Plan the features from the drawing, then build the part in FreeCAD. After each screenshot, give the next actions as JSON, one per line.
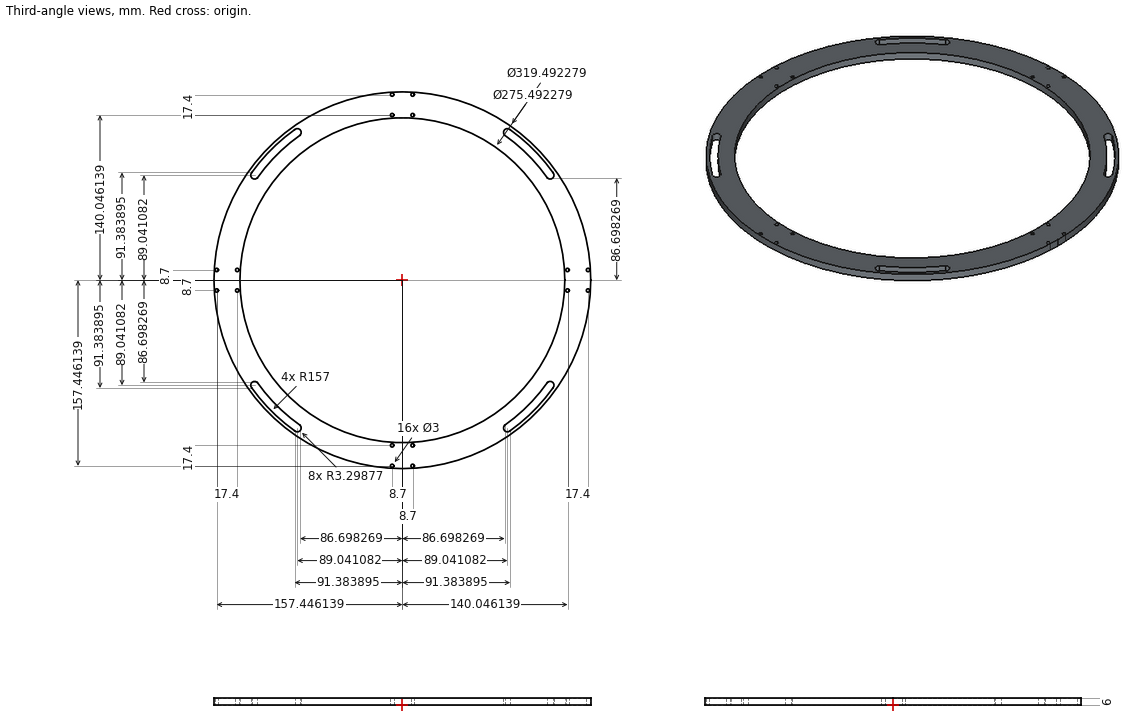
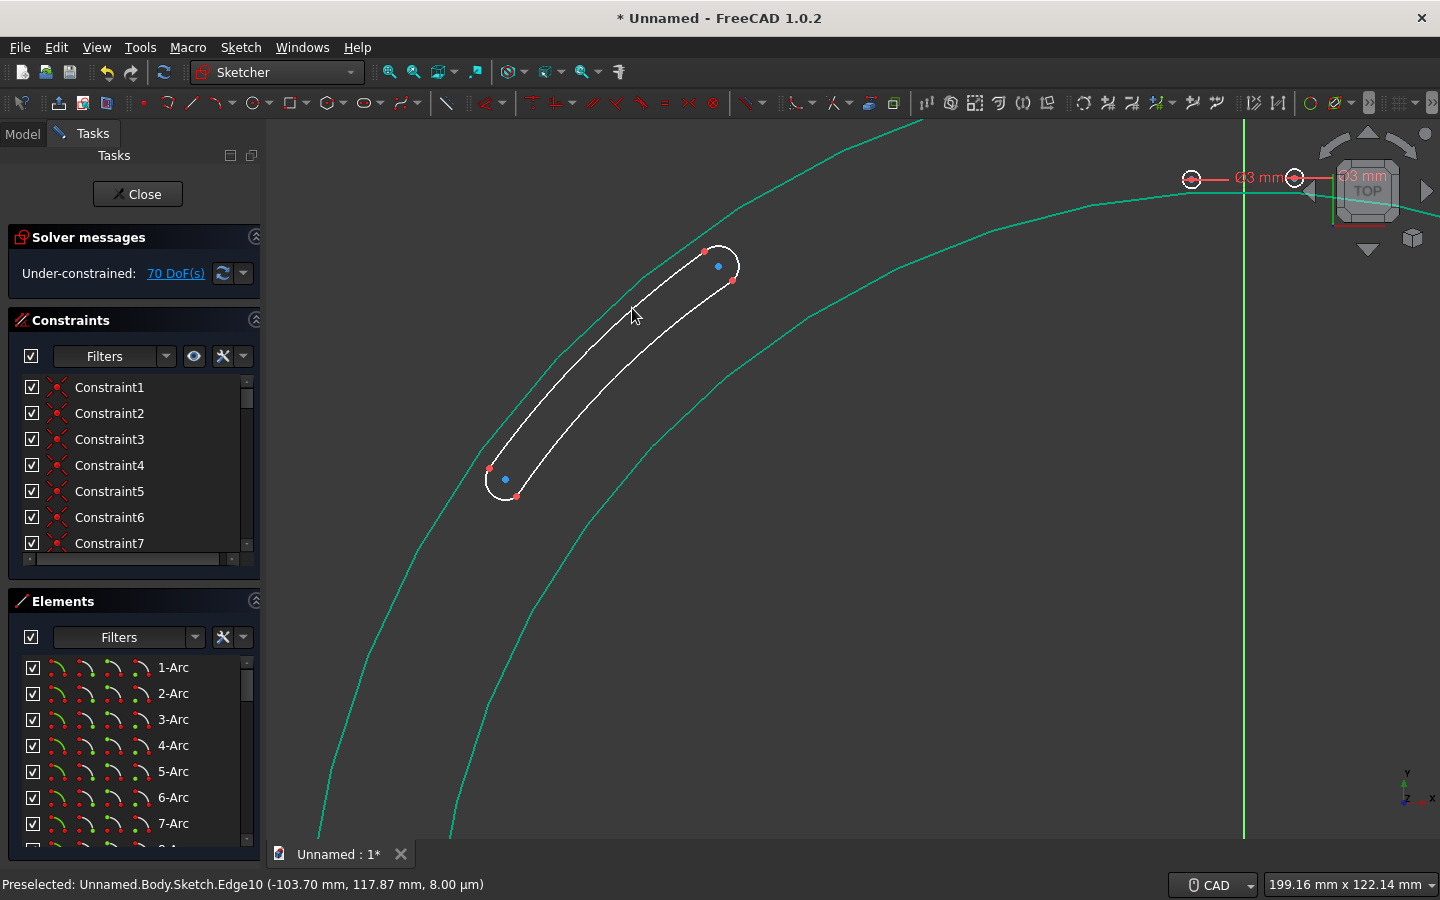
{"action": "left_click", "coordinate": [576, 339]}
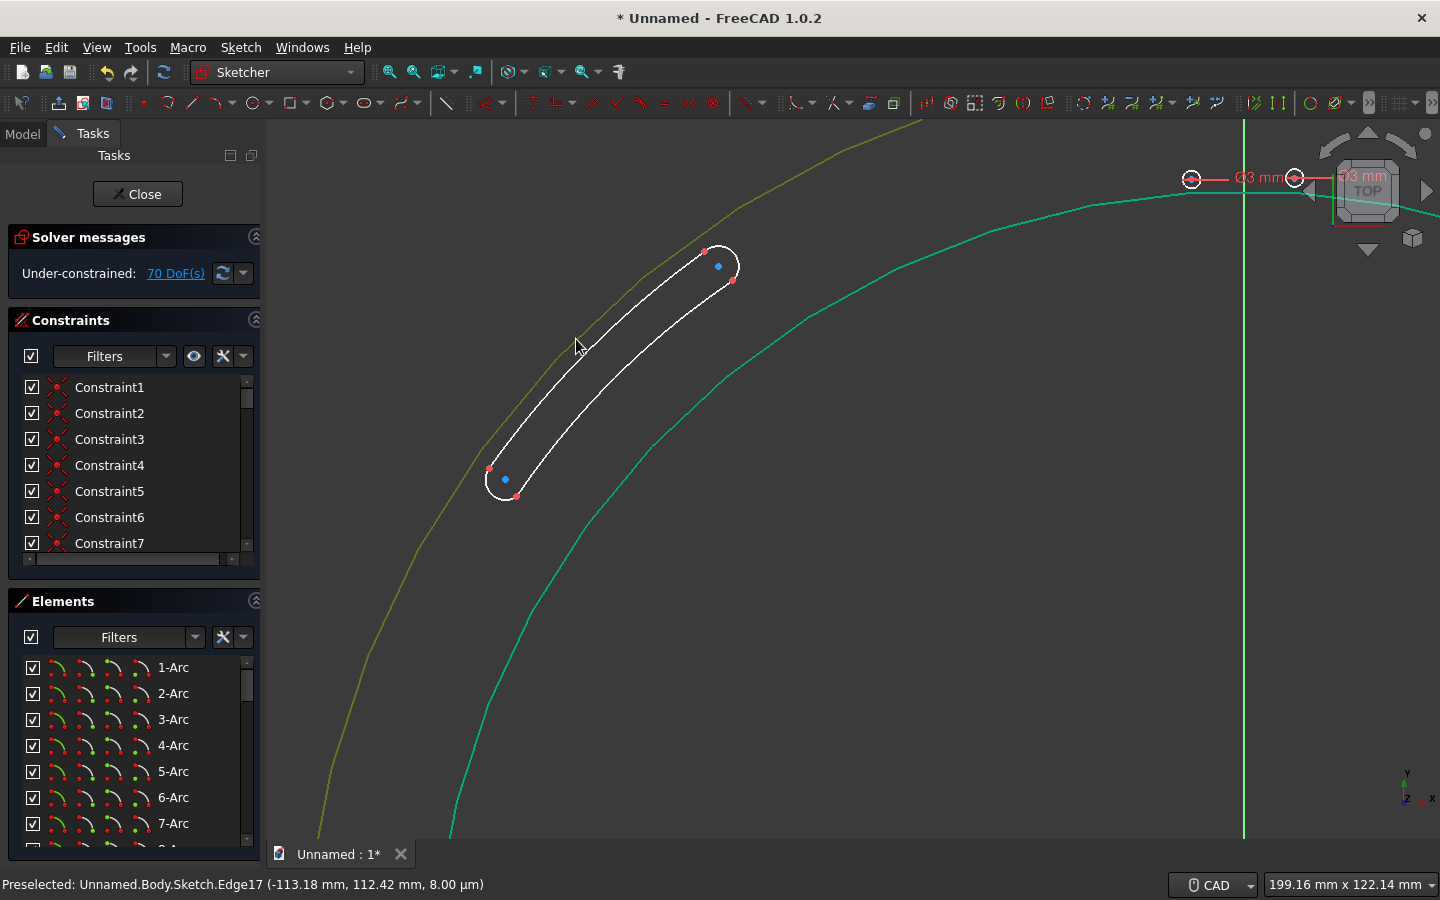
{"action": "left_click", "coordinate": [659, 337]}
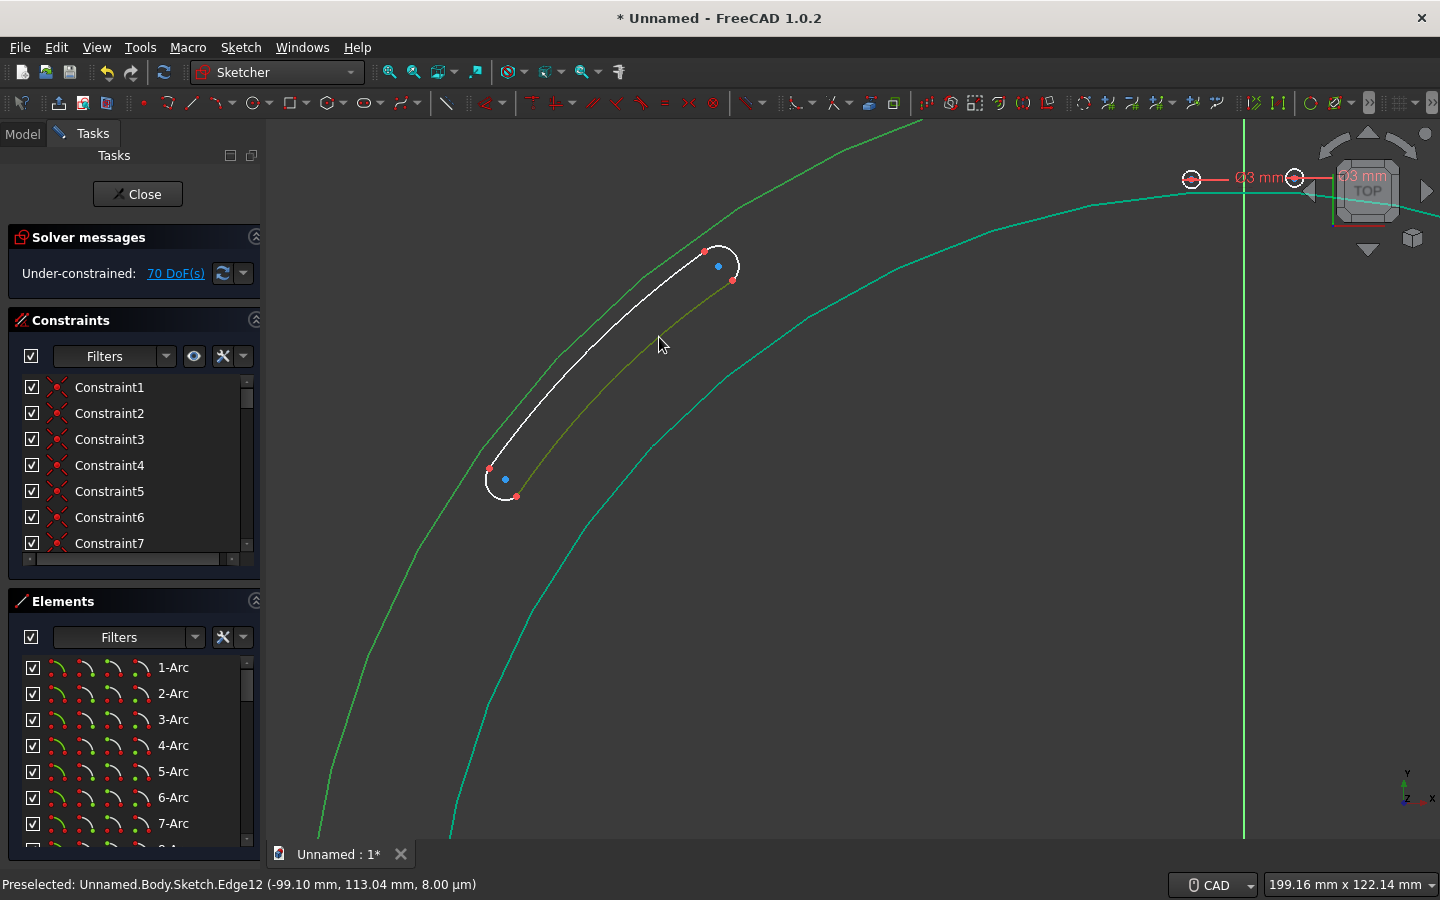
{"action": "left_click", "coordinate": [532, 104]}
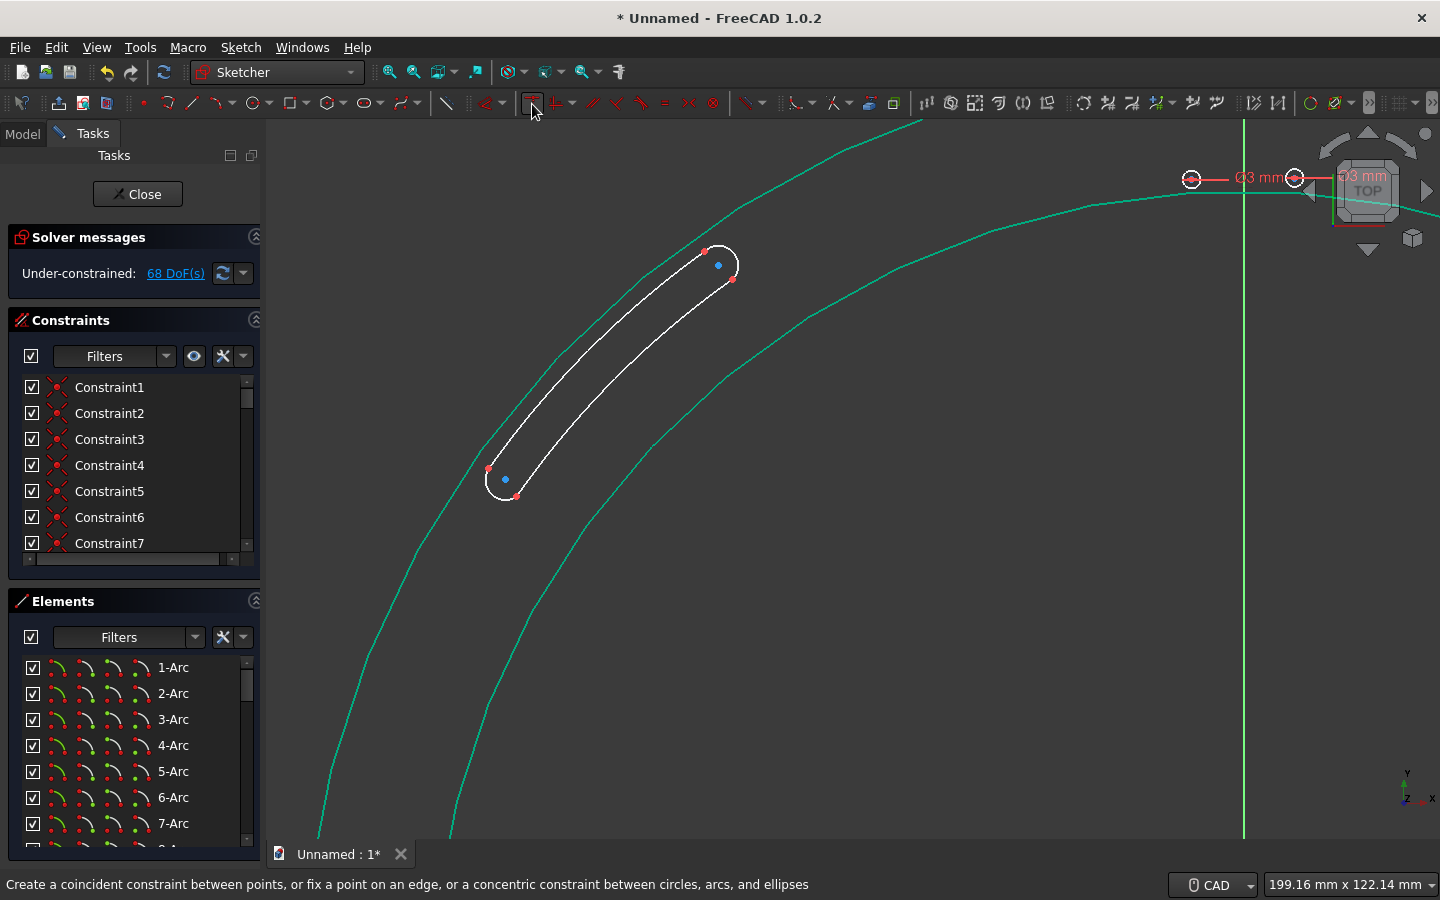
{"action": "left_click", "coordinate": [576, 339]}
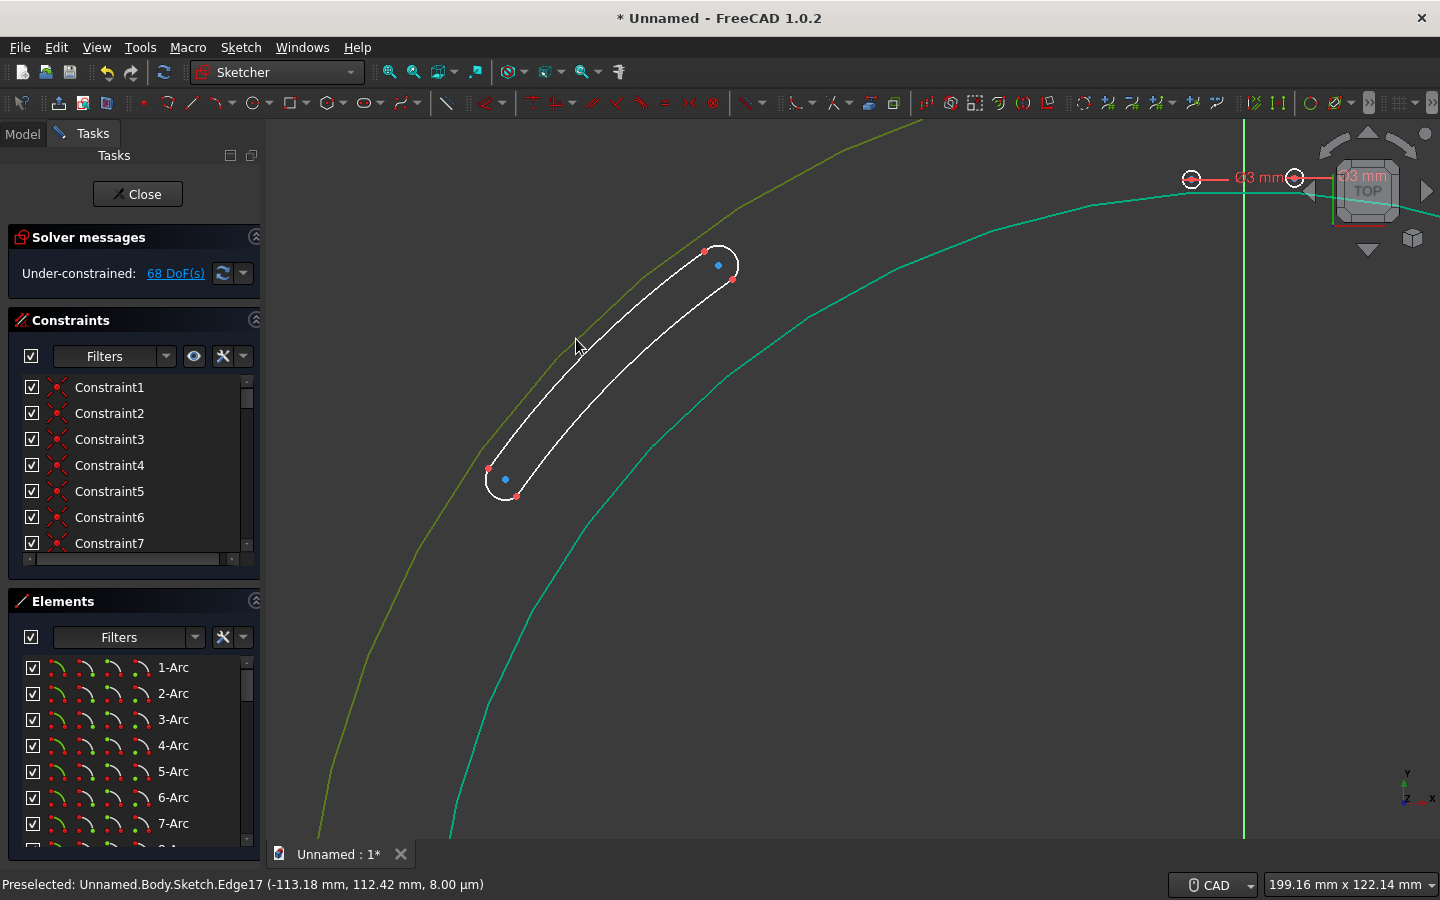
{"action": "scroll", "coordinate": [634, 307], "scroll_direction": "down", "scroll_amount": 7}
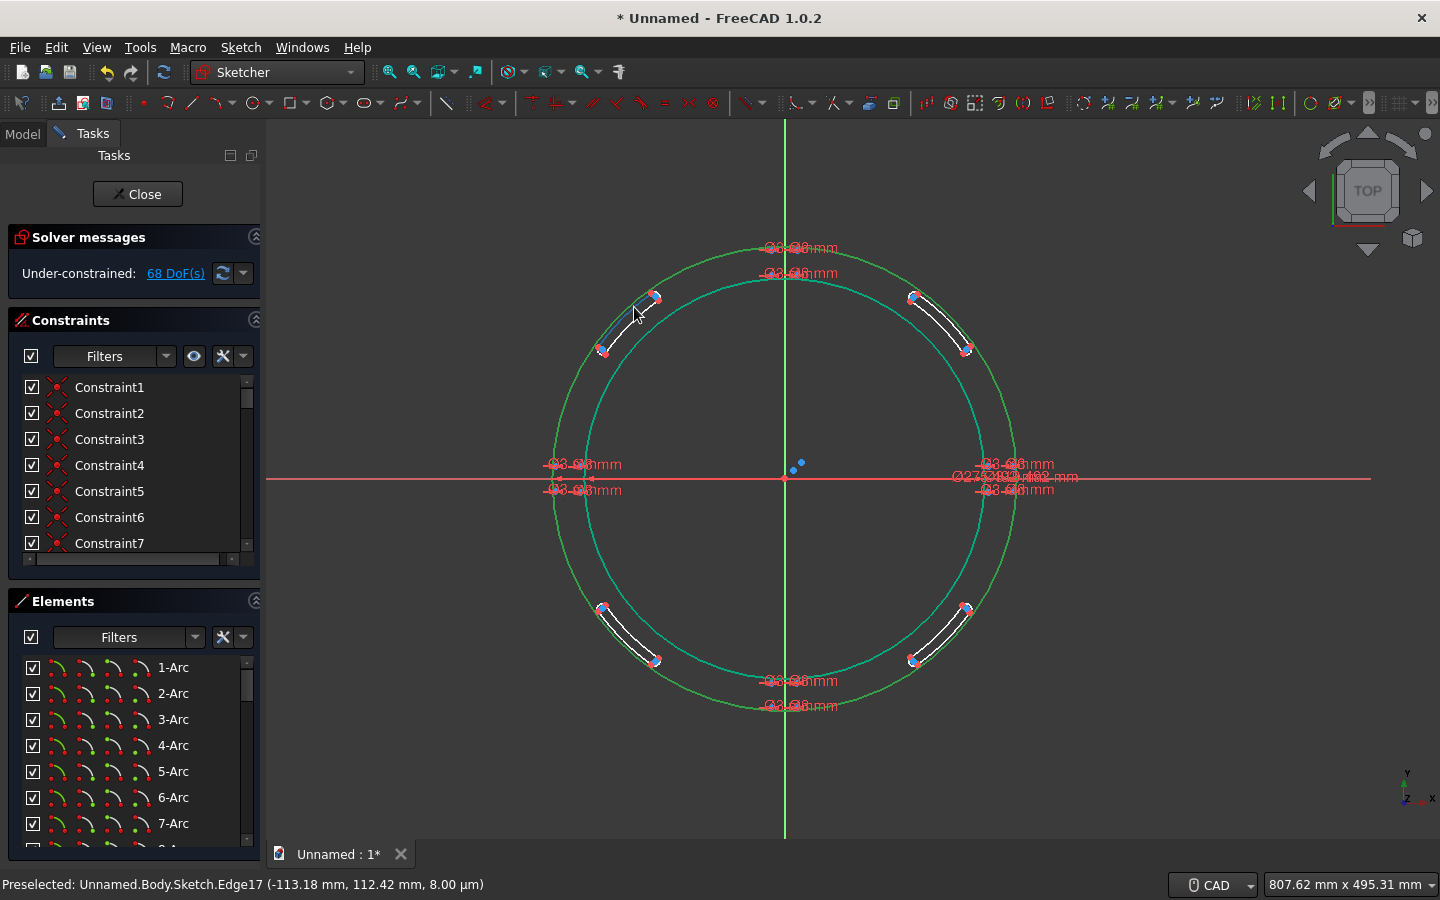
{"action": "scroll", "coordinate": [956, 329], "scroll_direction": "up", "scroll_amount": 7}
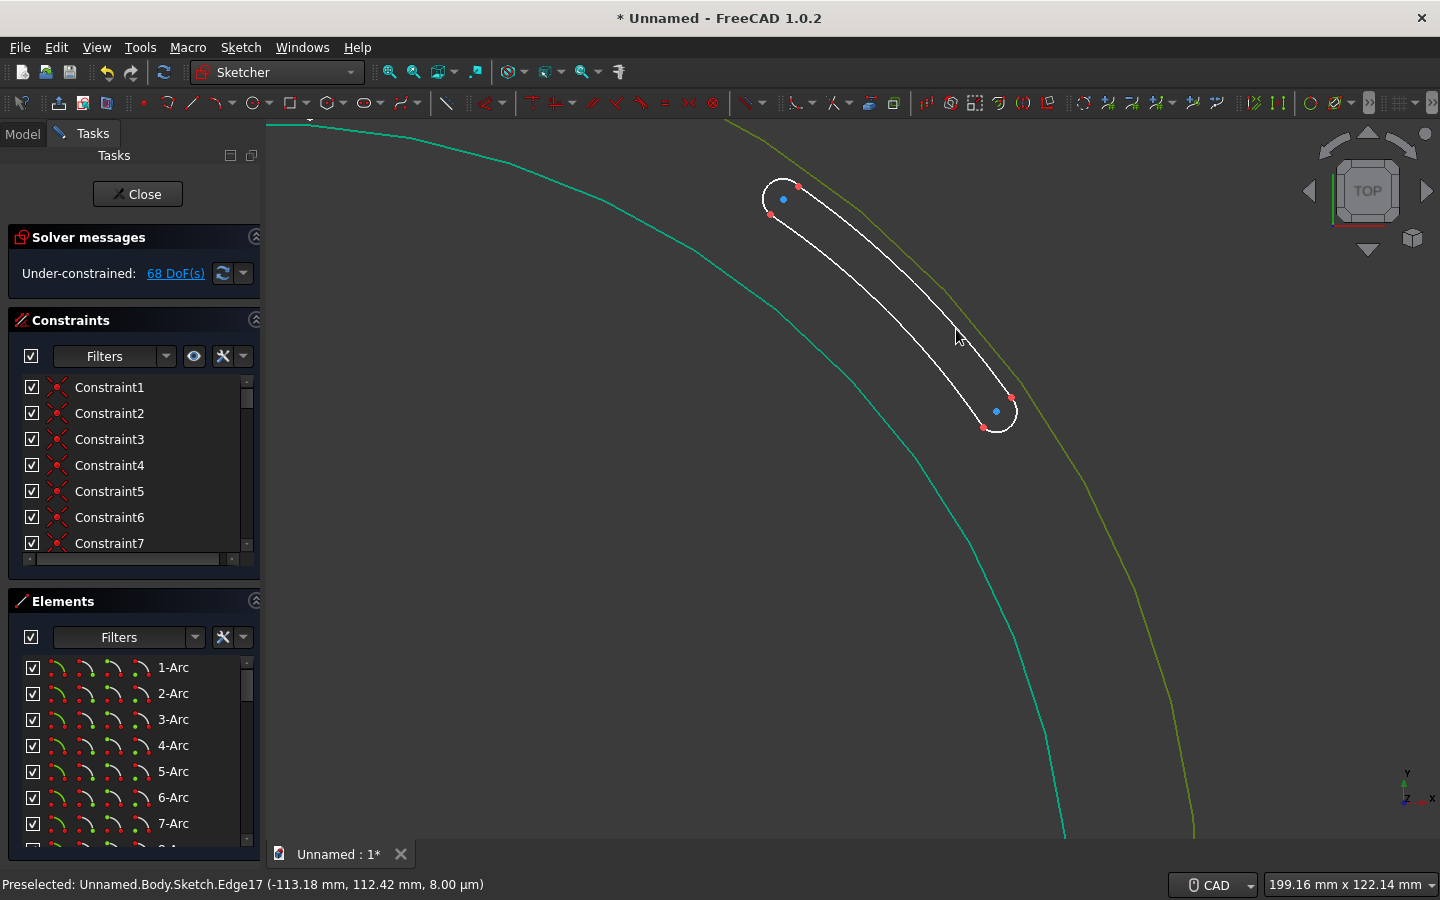
{"action": "left_click", "coordinate": [955, 327]}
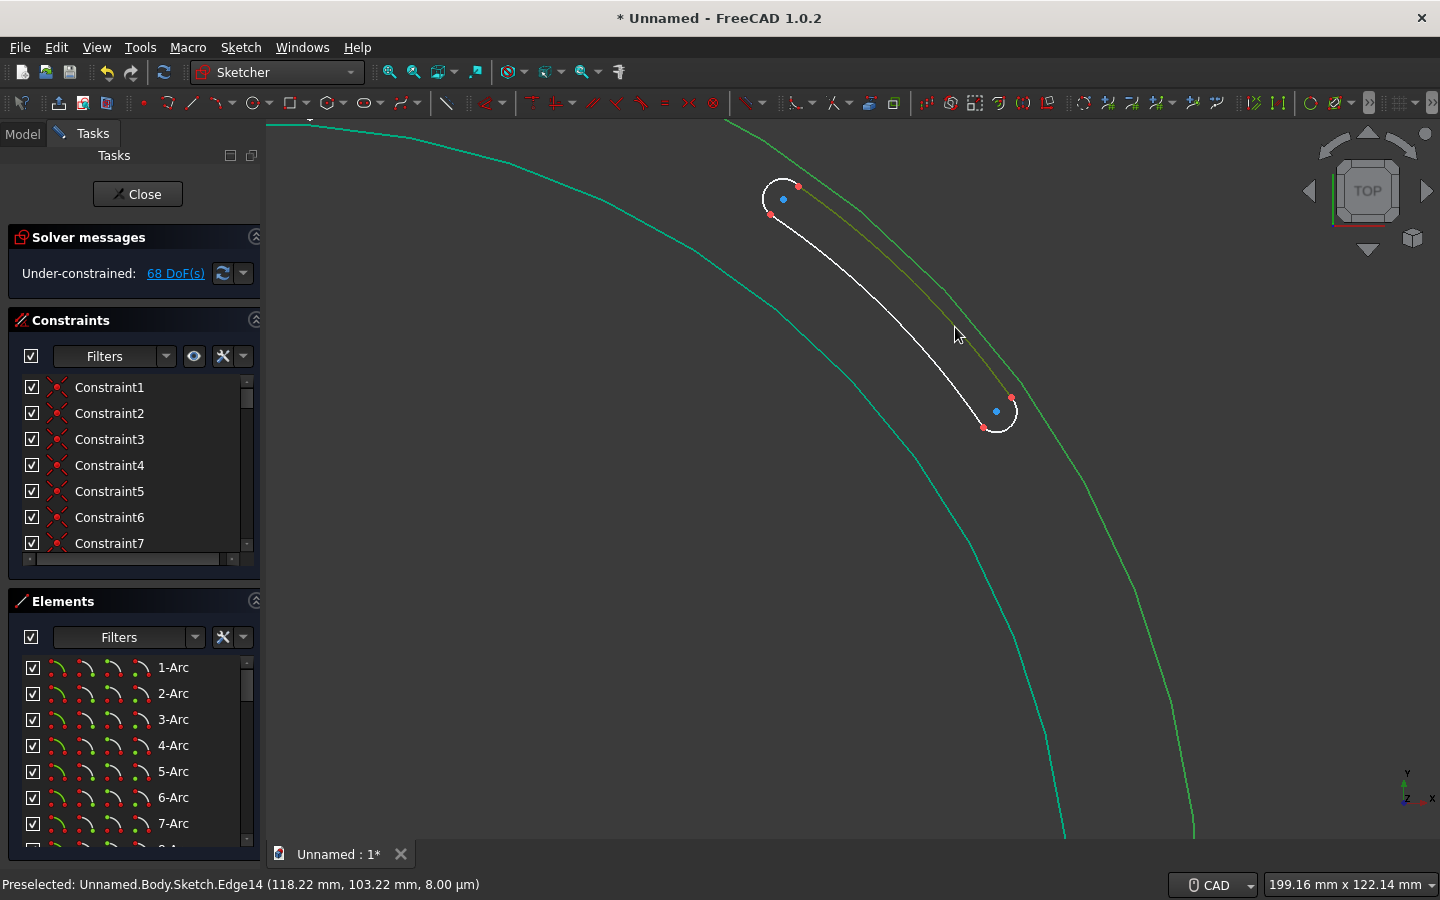
{"action": "key", "text": "c"}